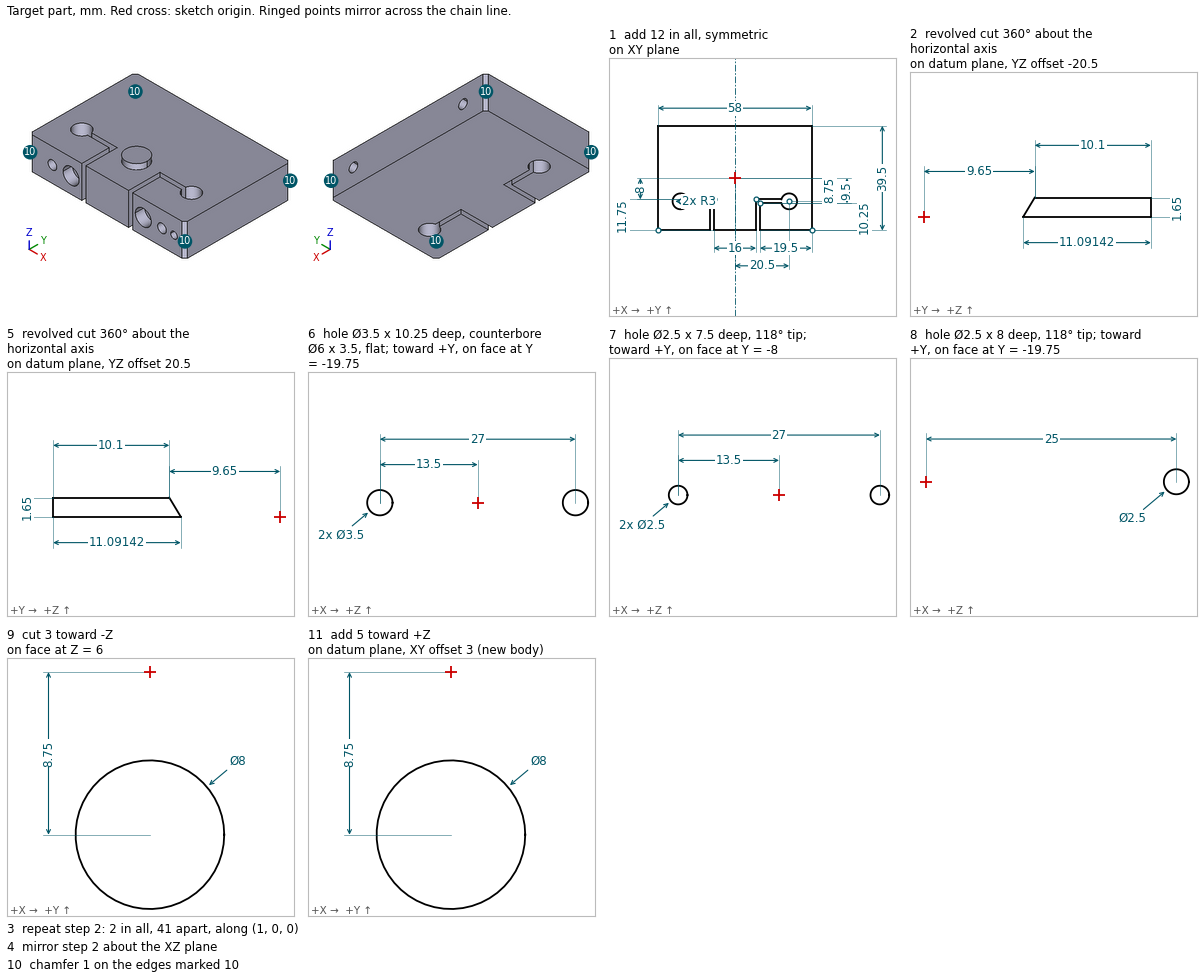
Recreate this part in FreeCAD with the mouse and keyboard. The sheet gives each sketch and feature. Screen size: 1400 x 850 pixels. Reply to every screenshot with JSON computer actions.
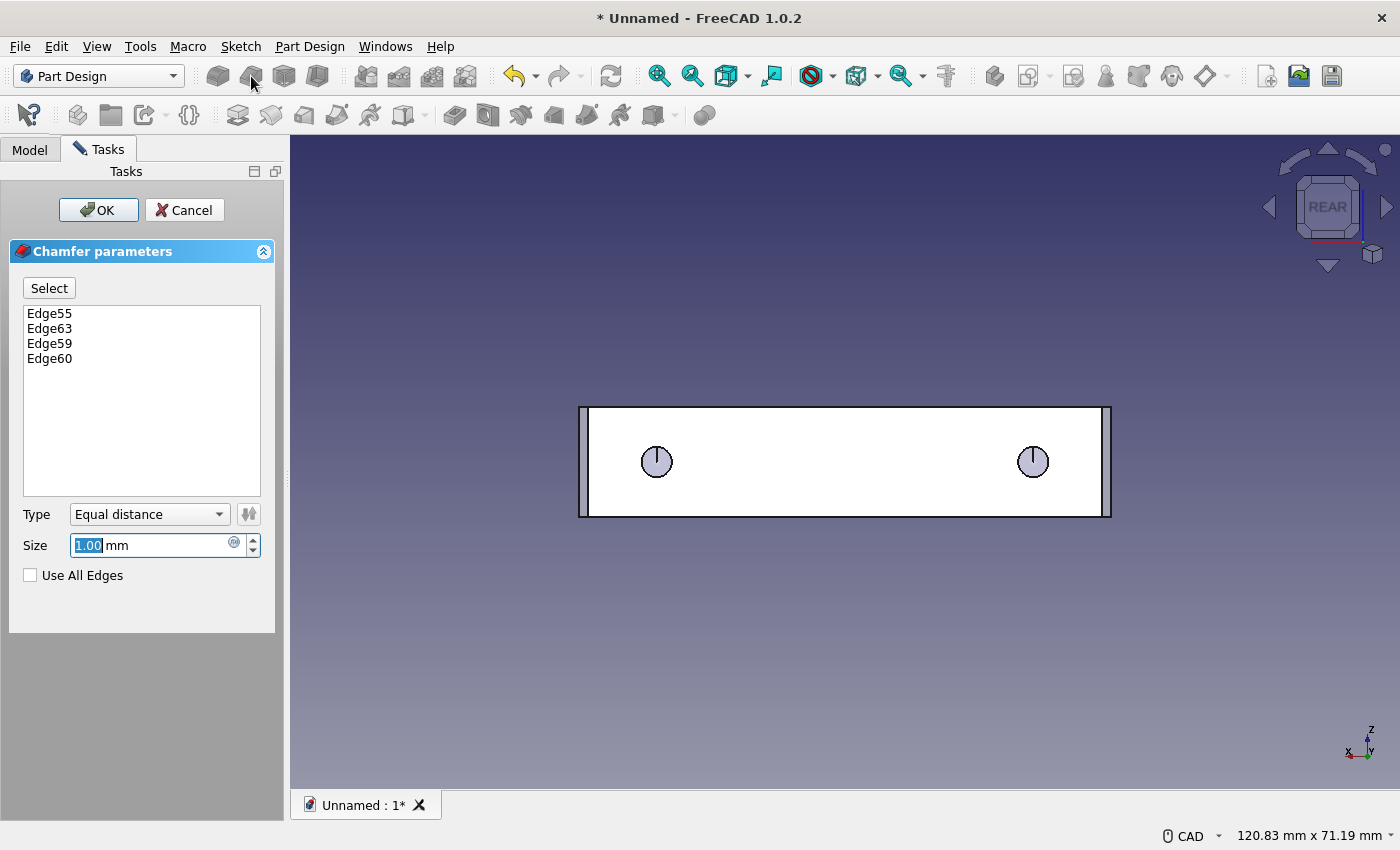
{"action": "type", "text": "1"}
{"action": "key", "text": "Tab"}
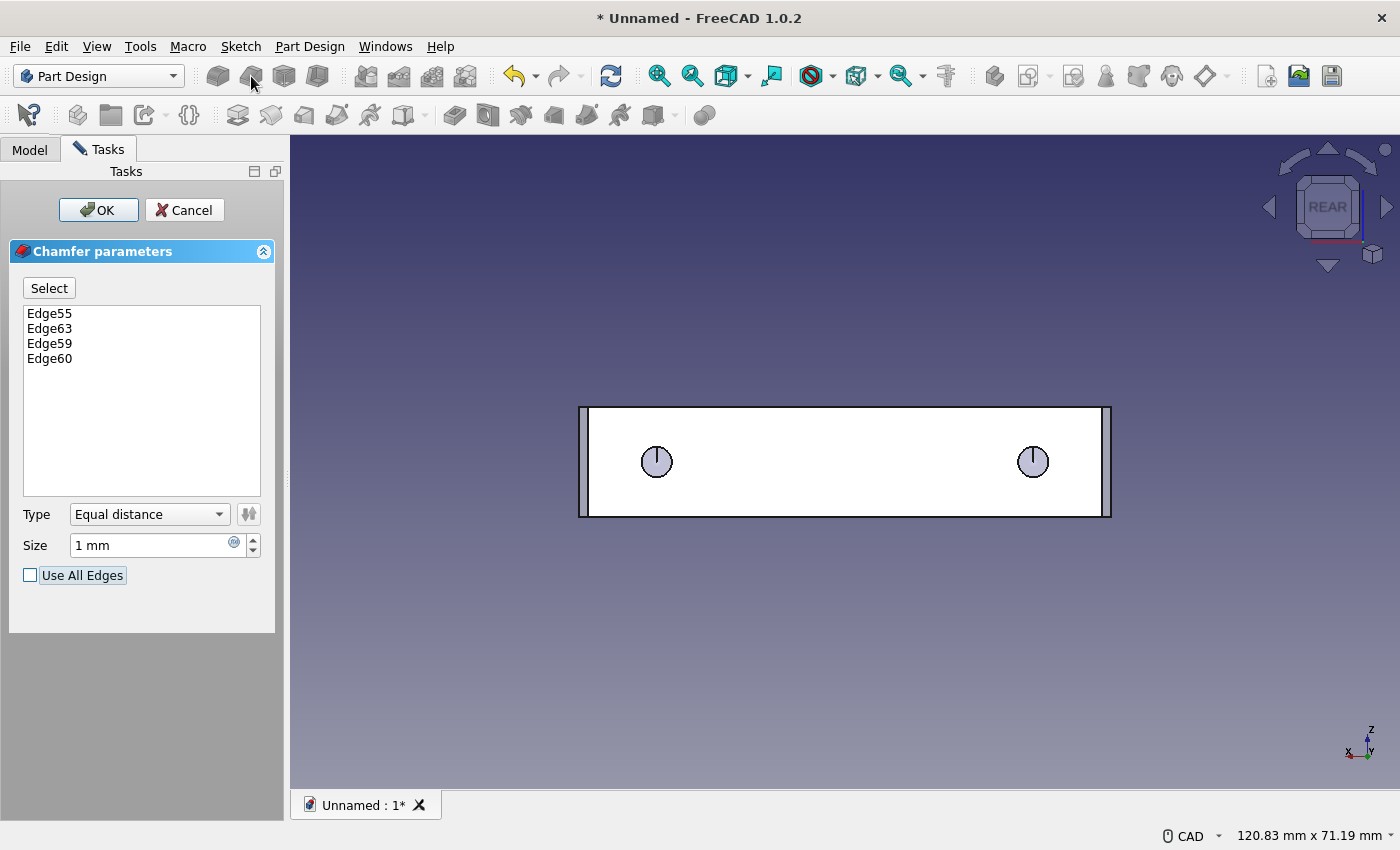
{"action": "left_click", "coordinate": [99, 210]}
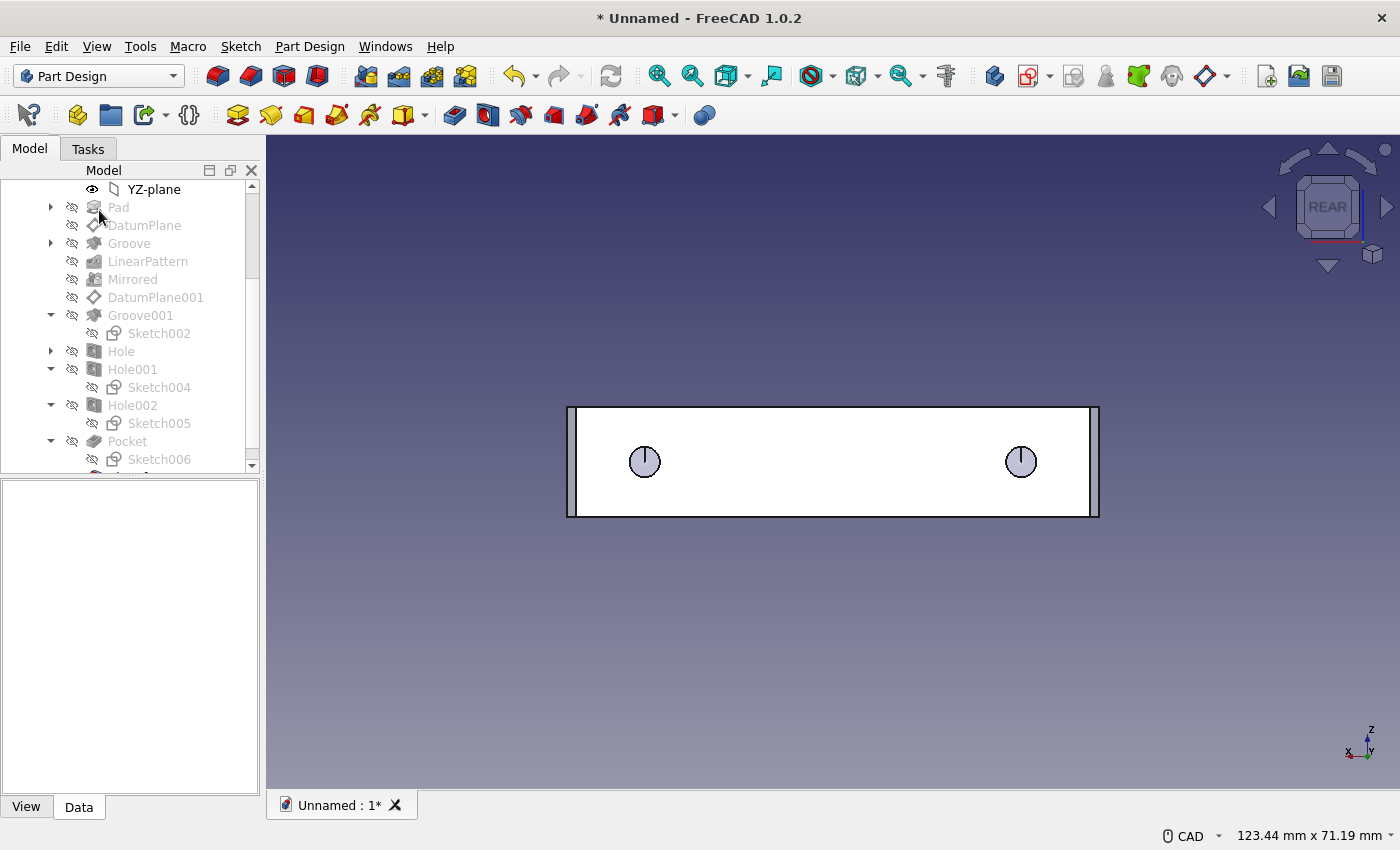
{"action": "left_click", "coordinate": [995, 76]}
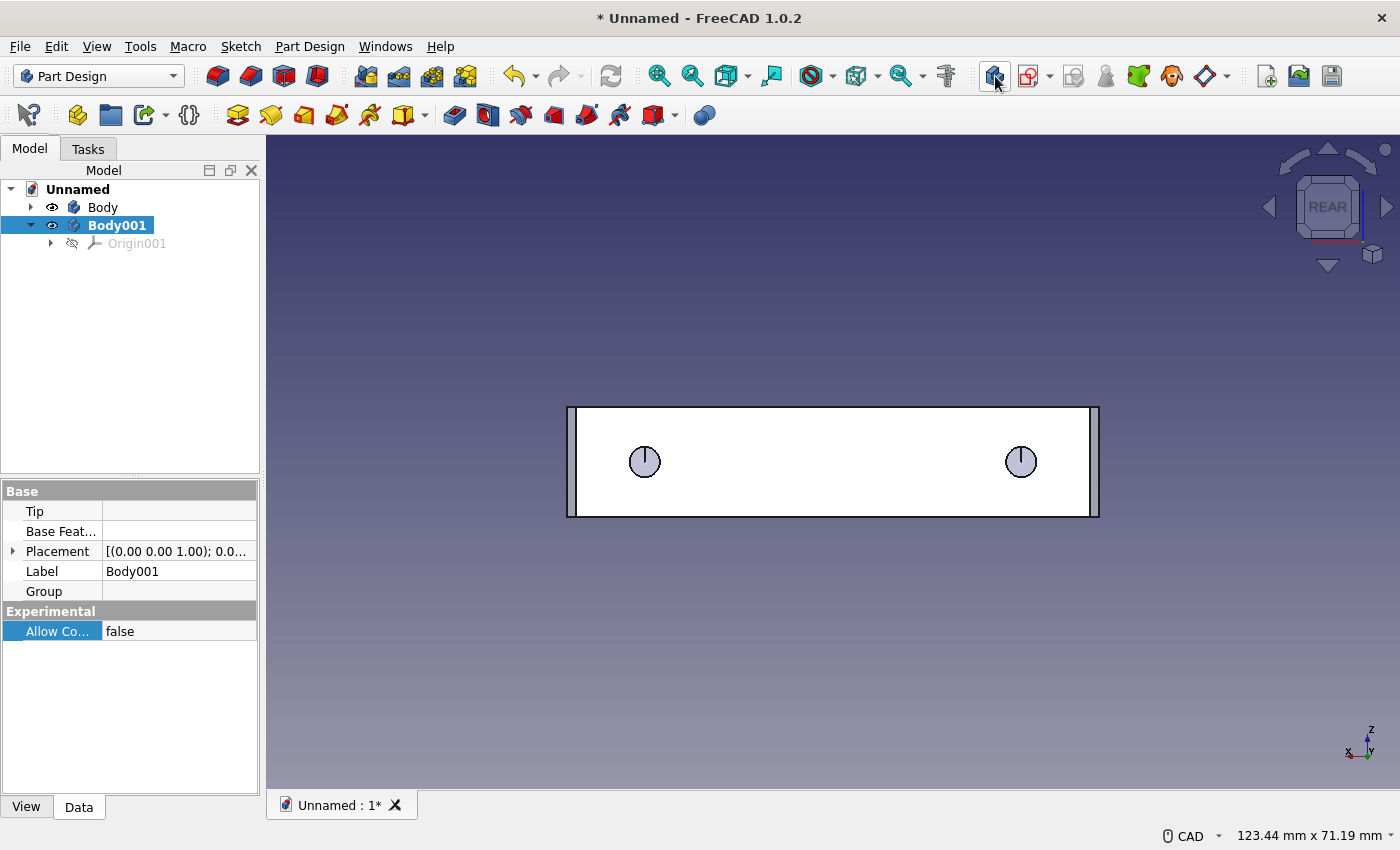
{"action": "left_click", "coordinate": [51, 243]}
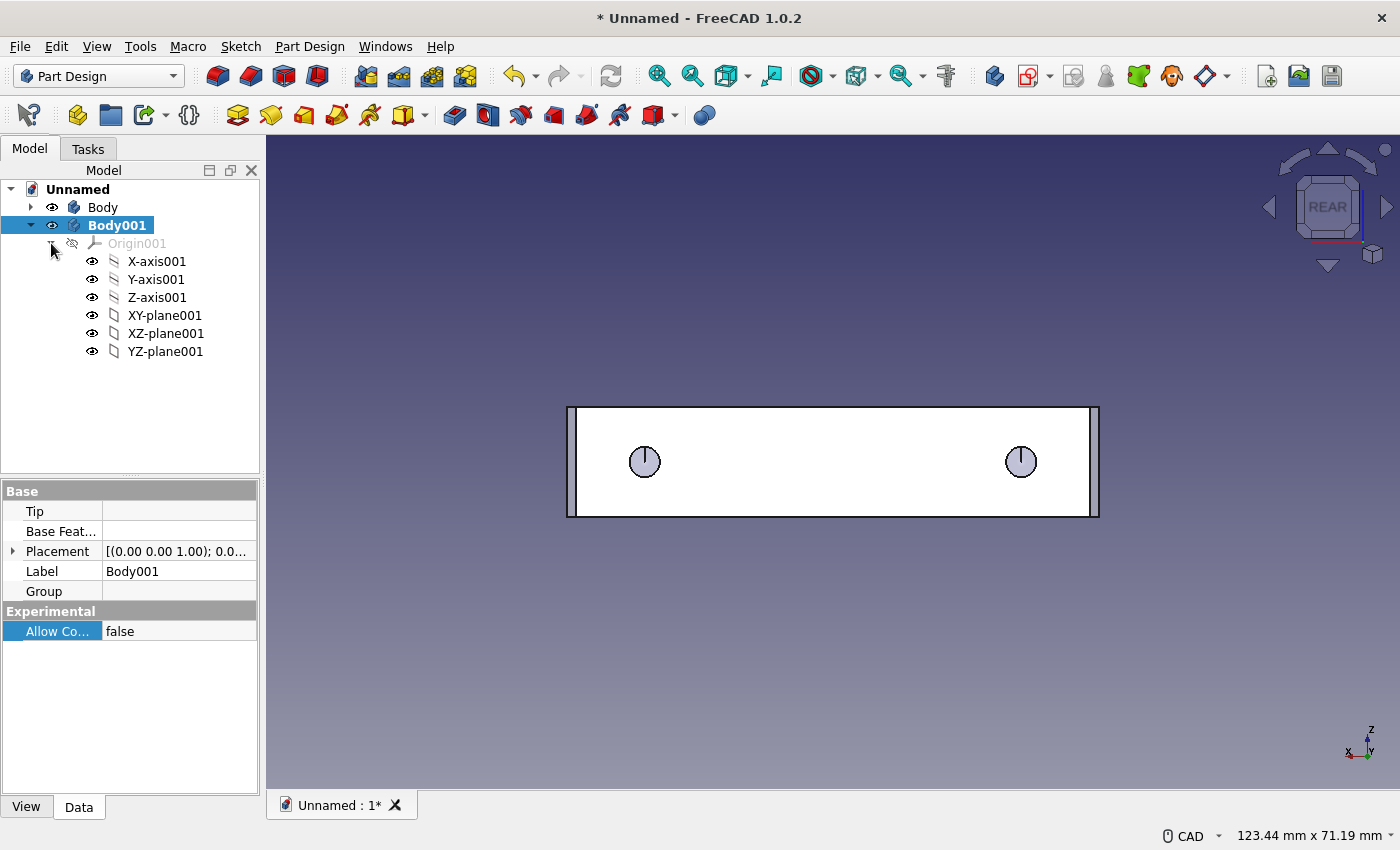
{"action": "left_click", "coordinate": [137, 315]}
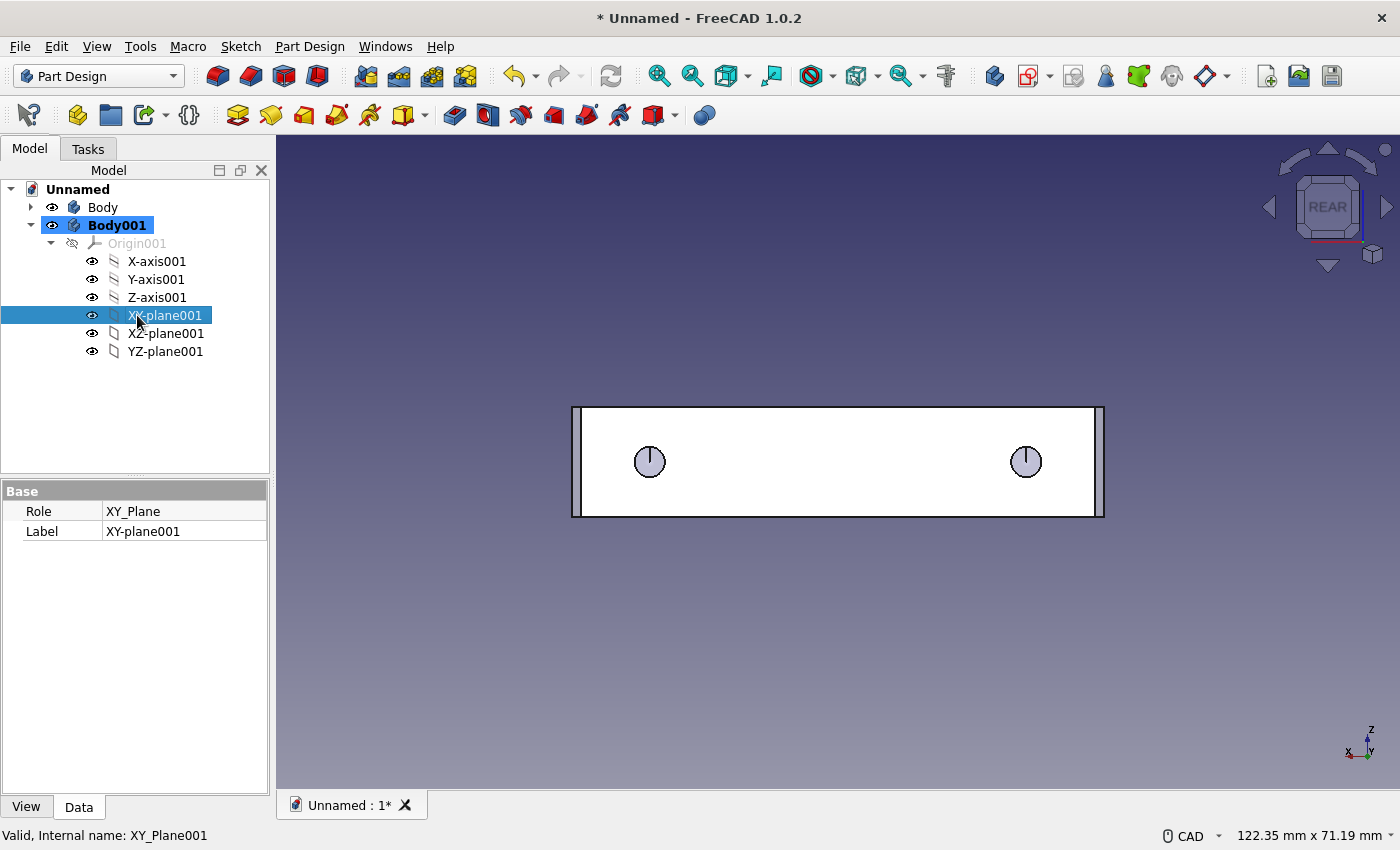
{"action": "left_click", "coordinate": [1204, 76]}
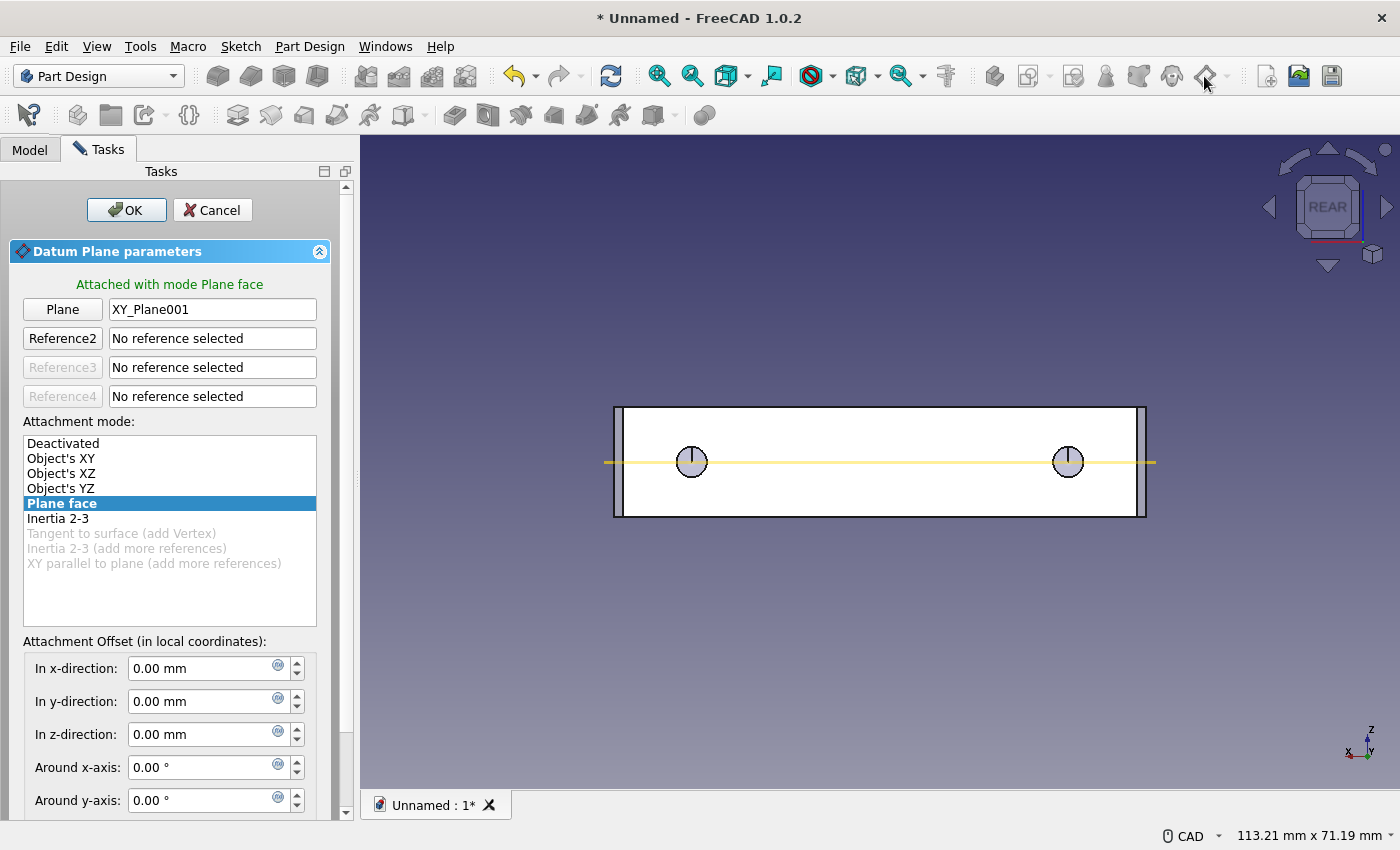
{"action": "triple_click", "coordinate": [210, 734]}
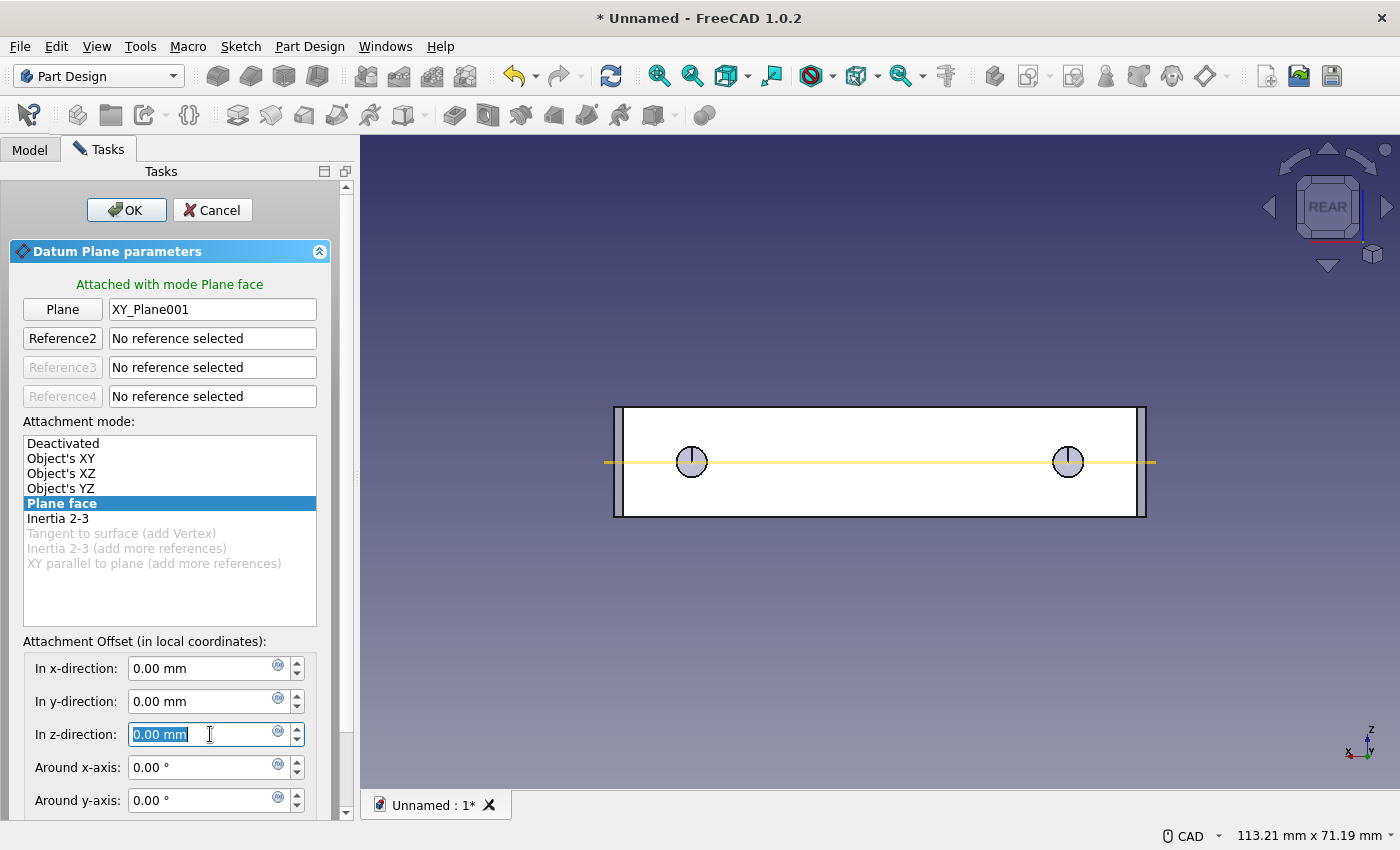
{"action": "type", "text": "3"}
{"action": "key", "text": "Tab"}